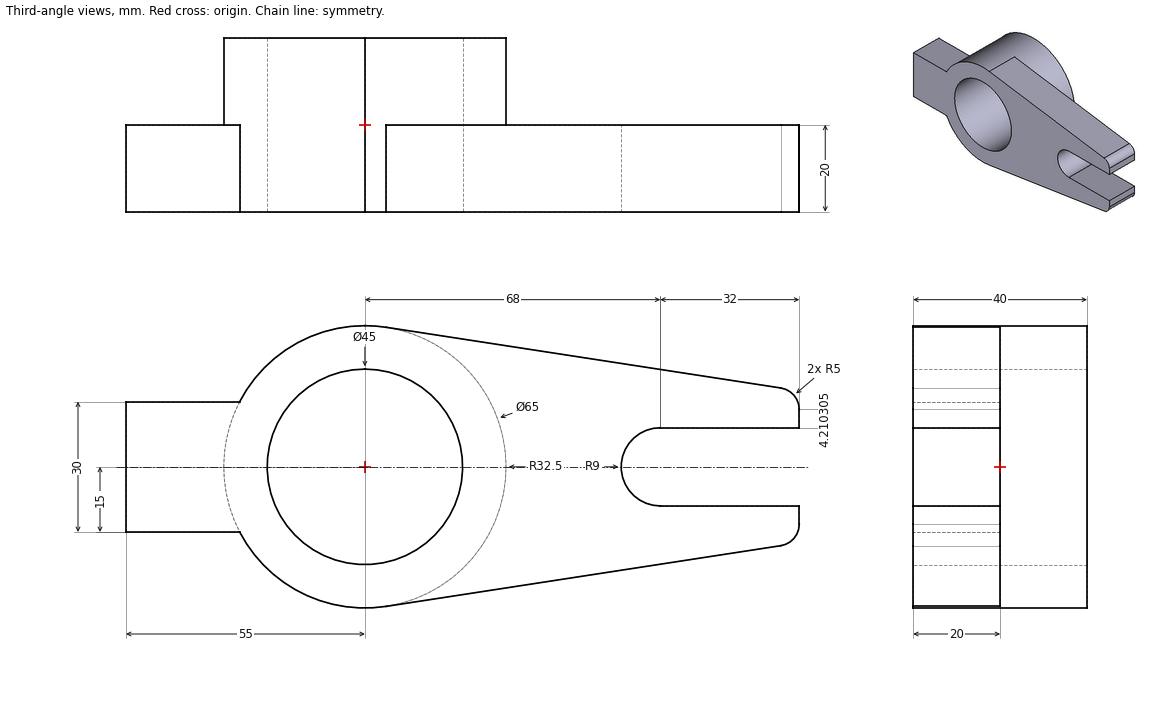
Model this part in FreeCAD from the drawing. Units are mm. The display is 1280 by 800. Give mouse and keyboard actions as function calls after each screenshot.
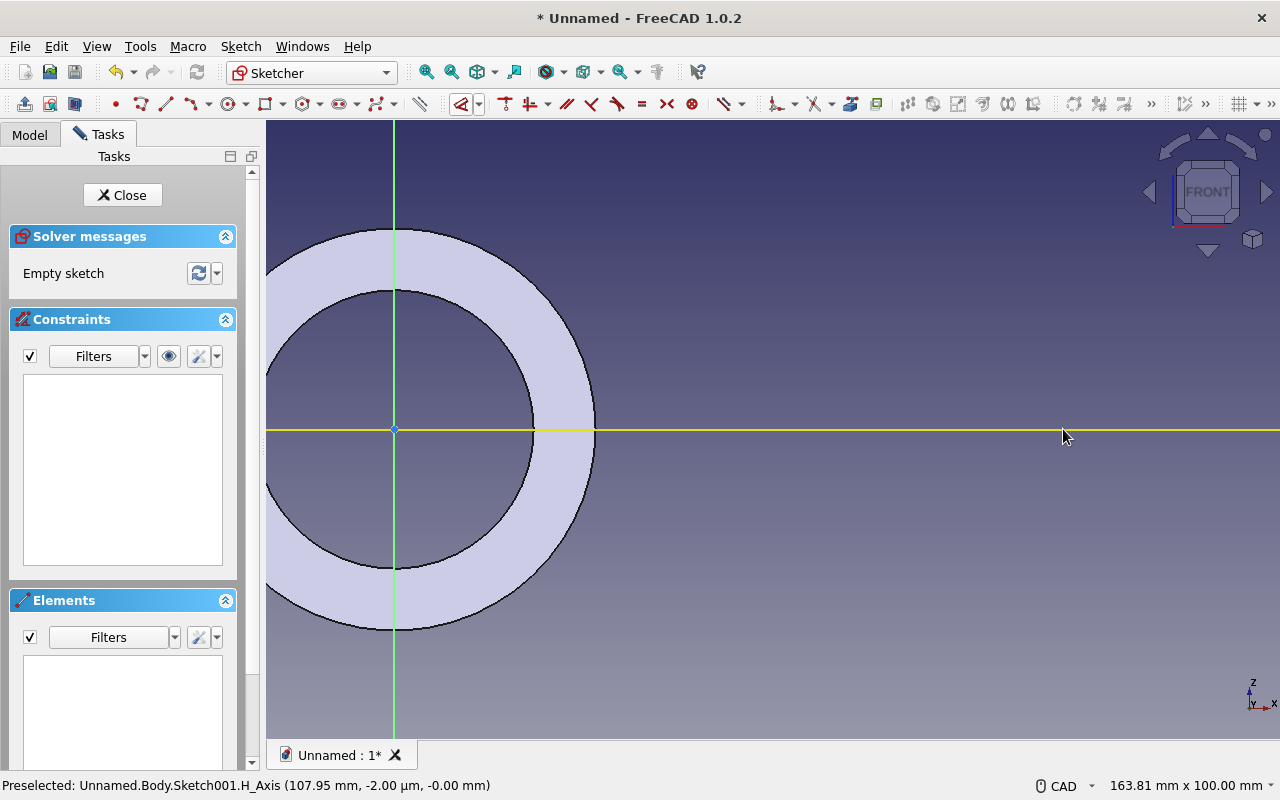
key(g)
key(l)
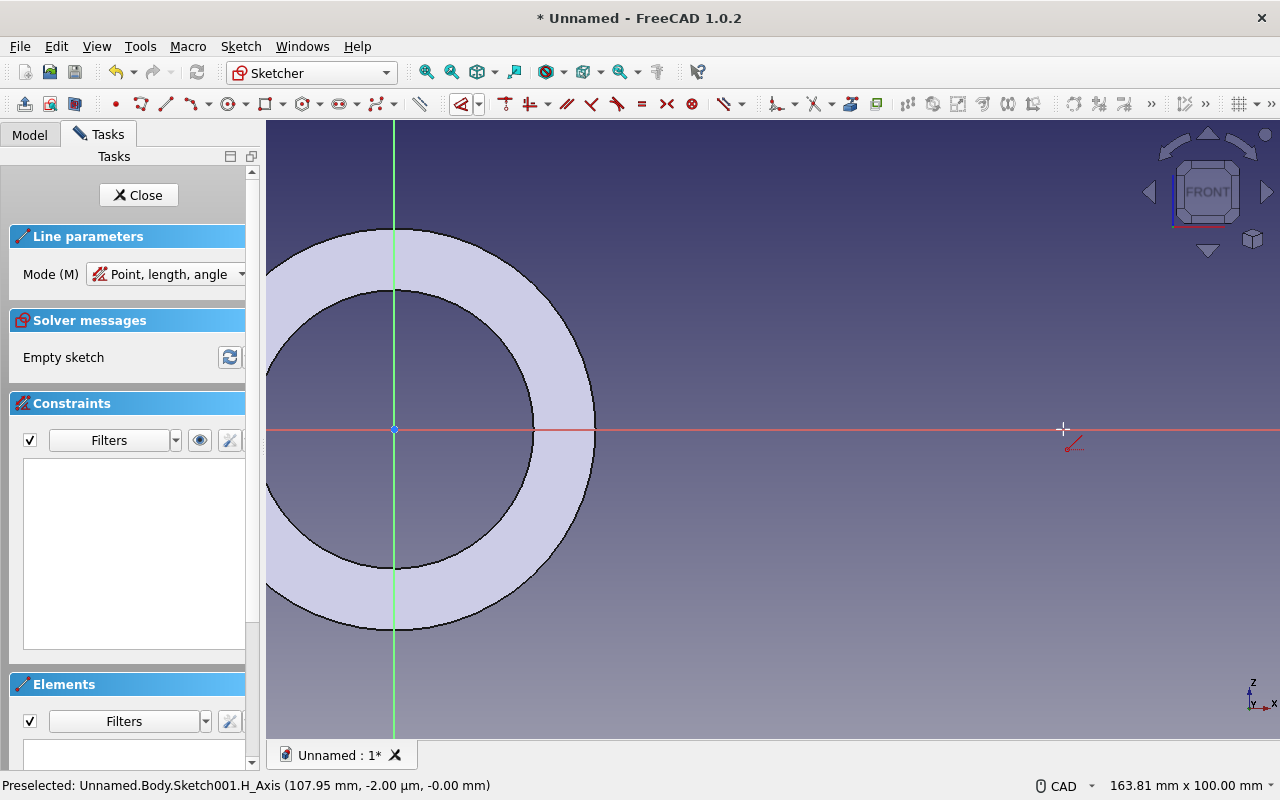
click(987, 542)
click(425, 628)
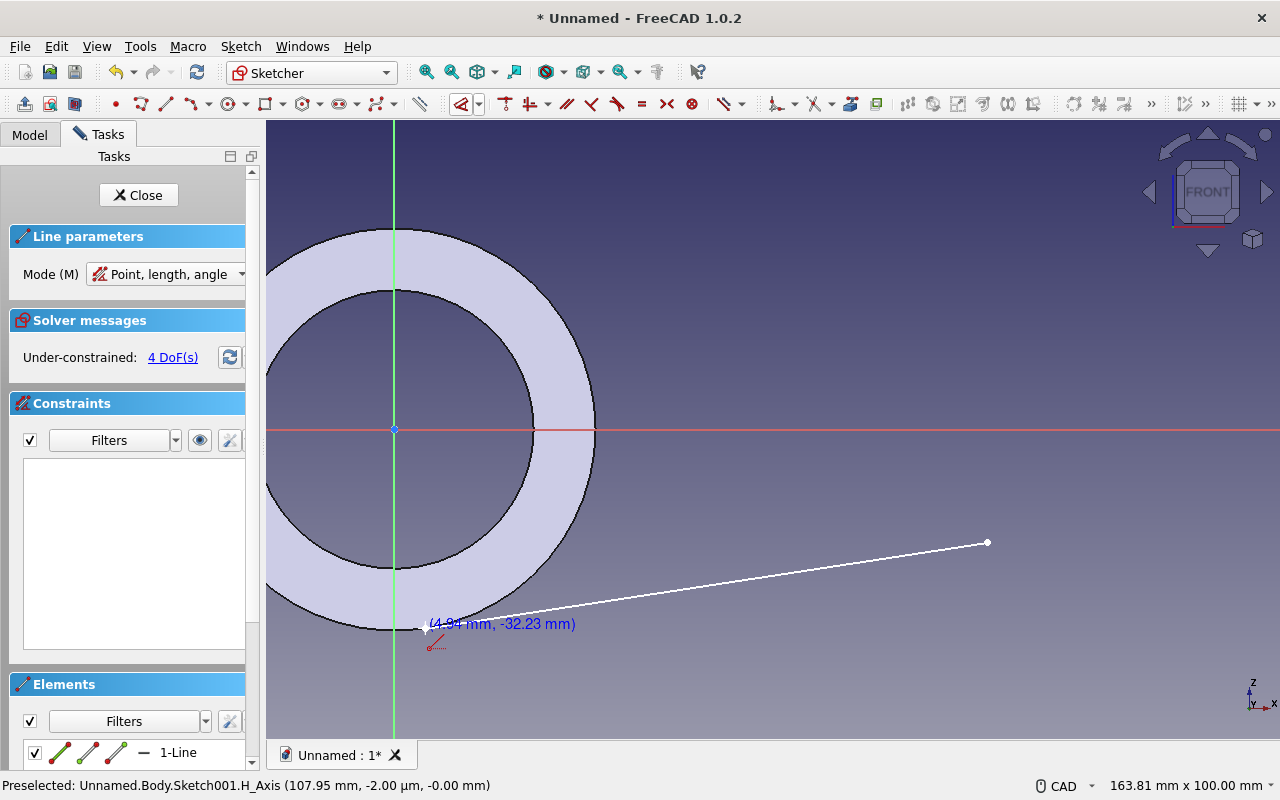
click(425, 231)
click(987, 317)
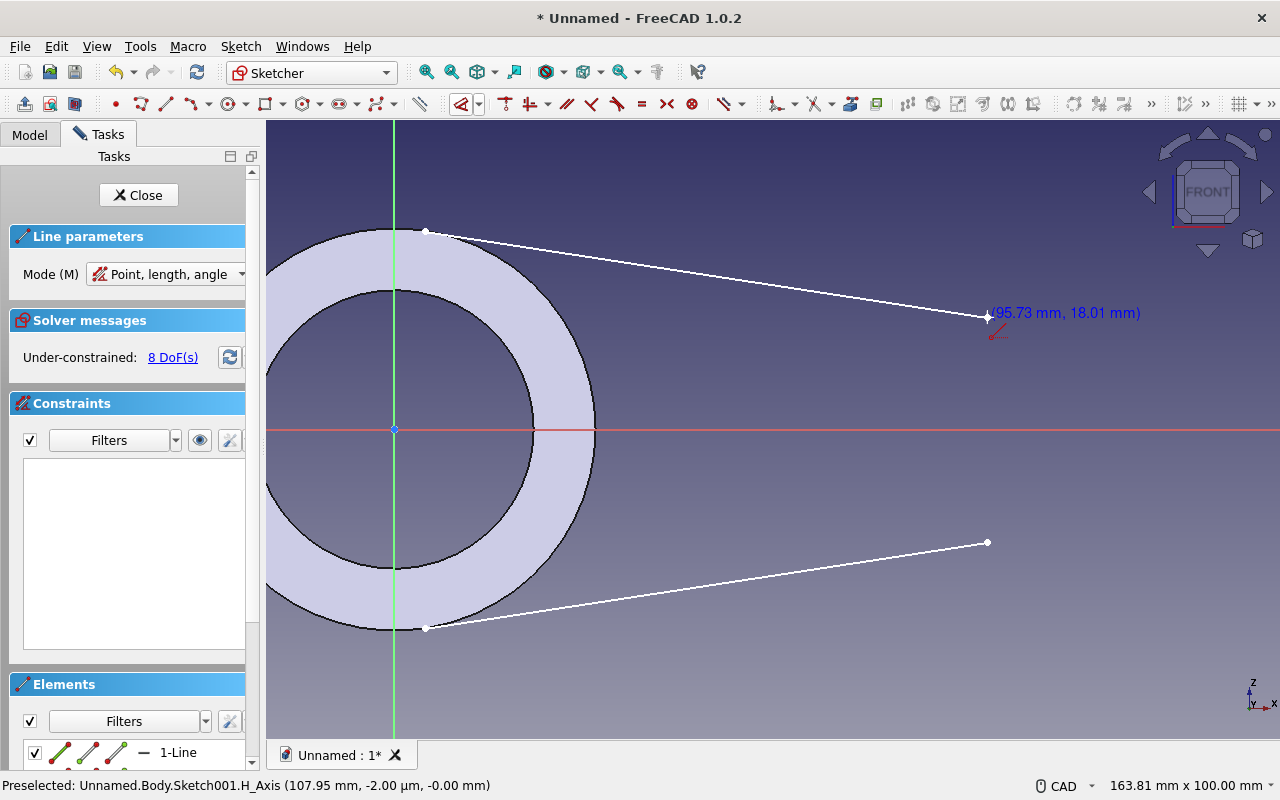
key(g)
key(m)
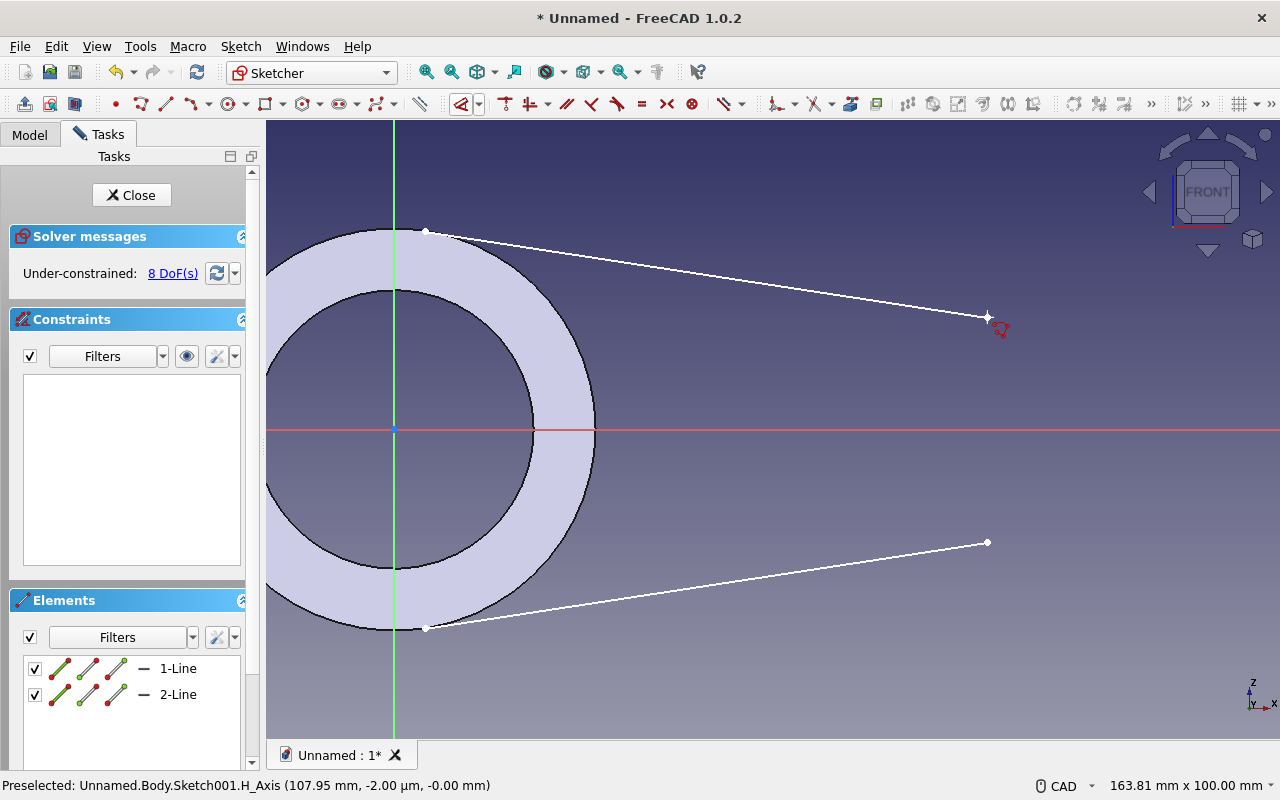
click(1013, 348)
click(1013, 374)
click(815, 374)
right_click(815, 374)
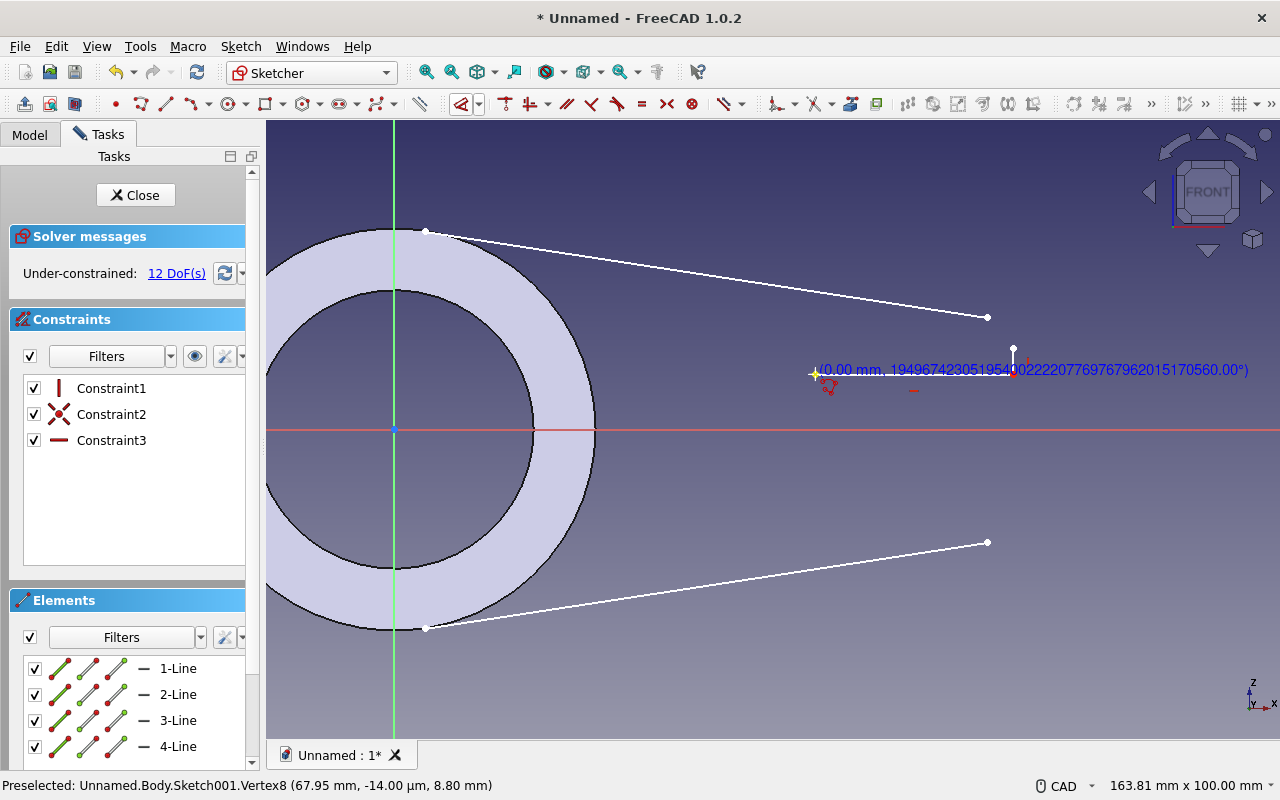
click(815, 485)
click(1013, 485)
click(1013, 511)
right_click(1013, 511)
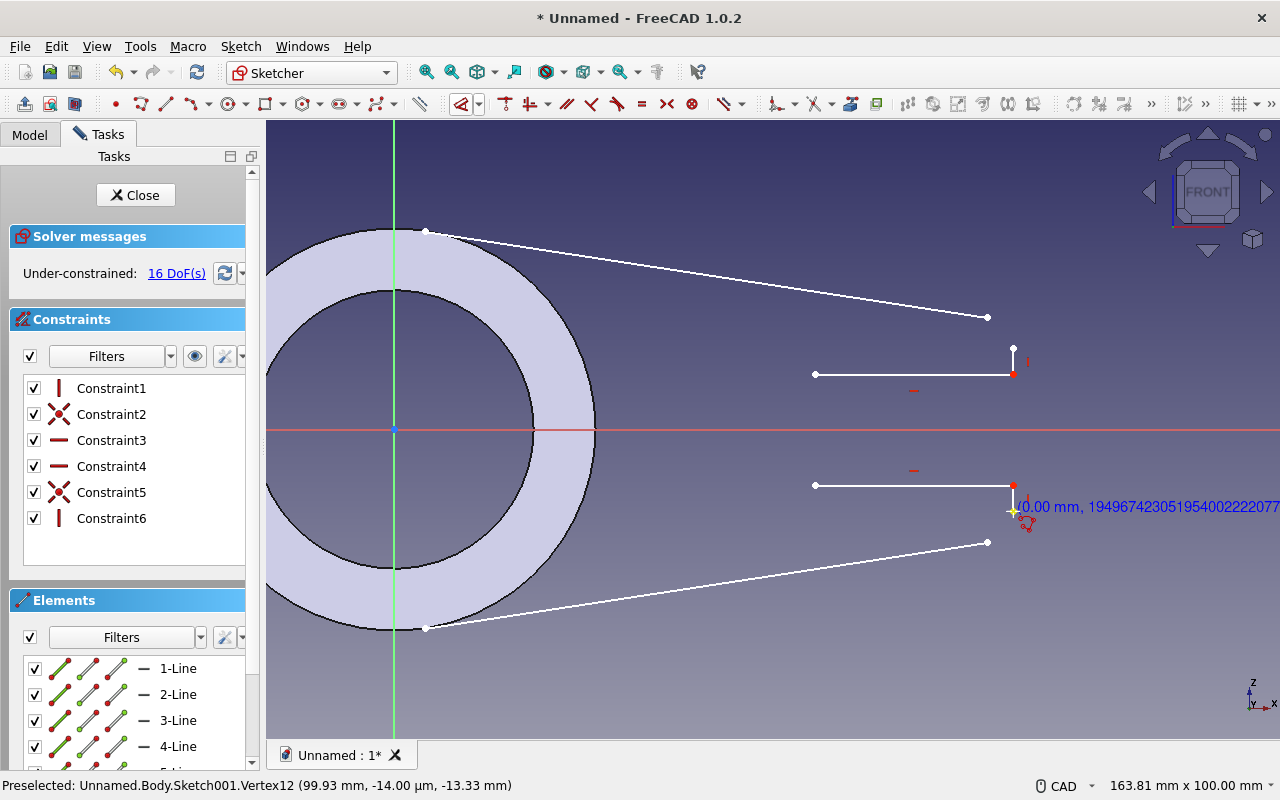
key(g)
key(3)
key(a)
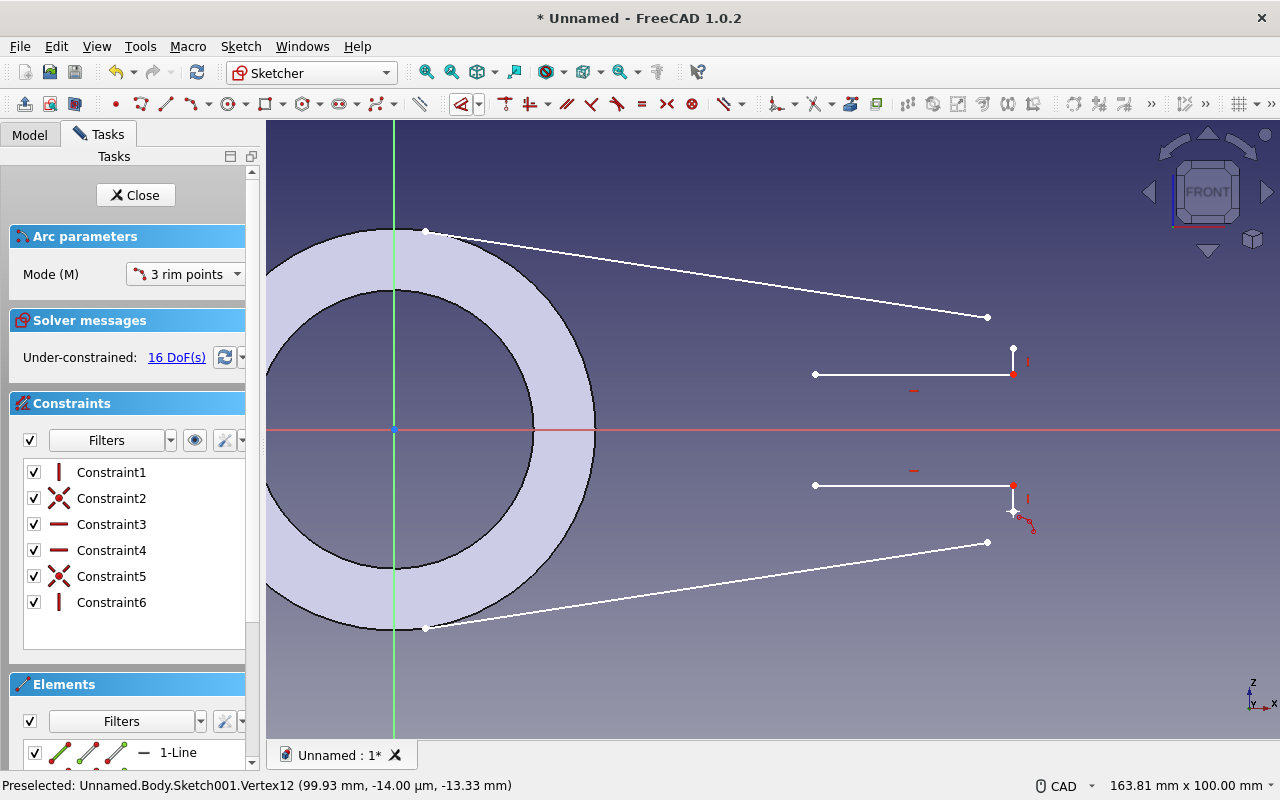
click(425, 629)
click(425, 232)
click(588, 486)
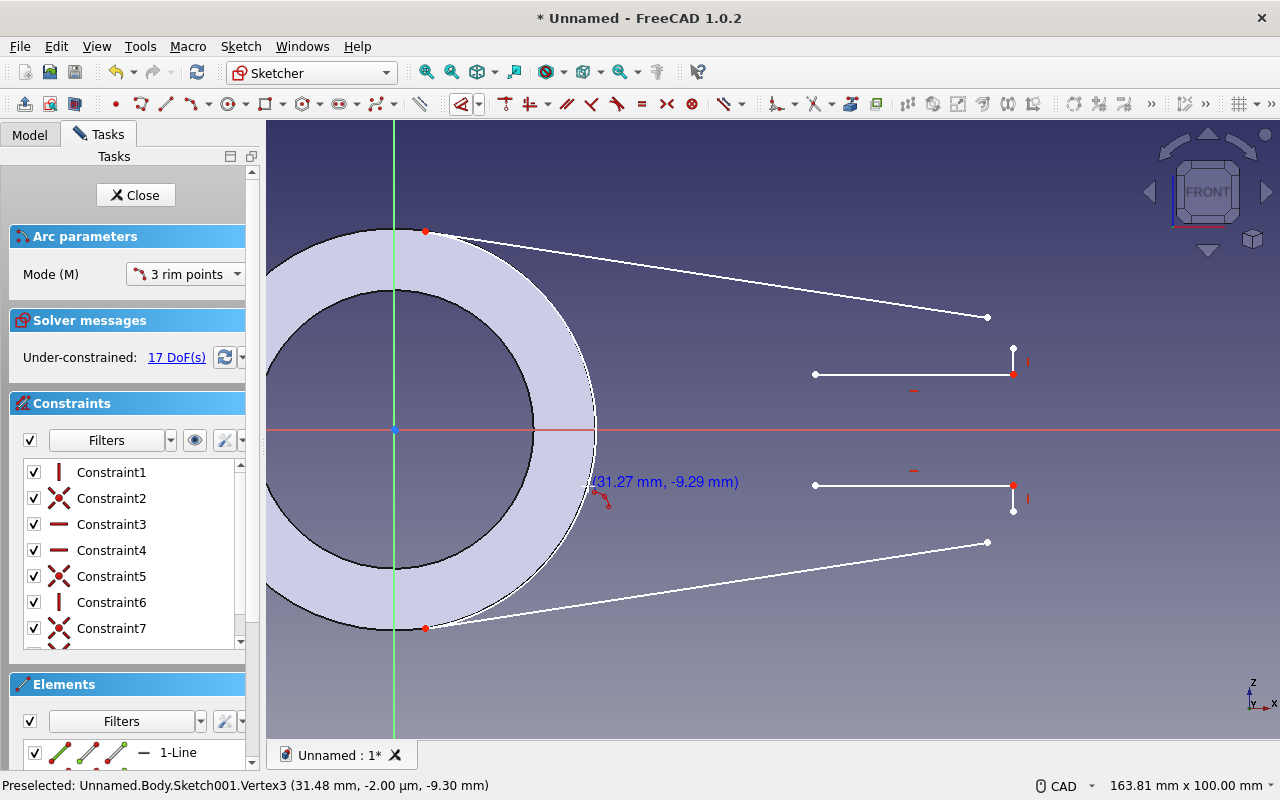
click(987, 318)
click(1013, 349)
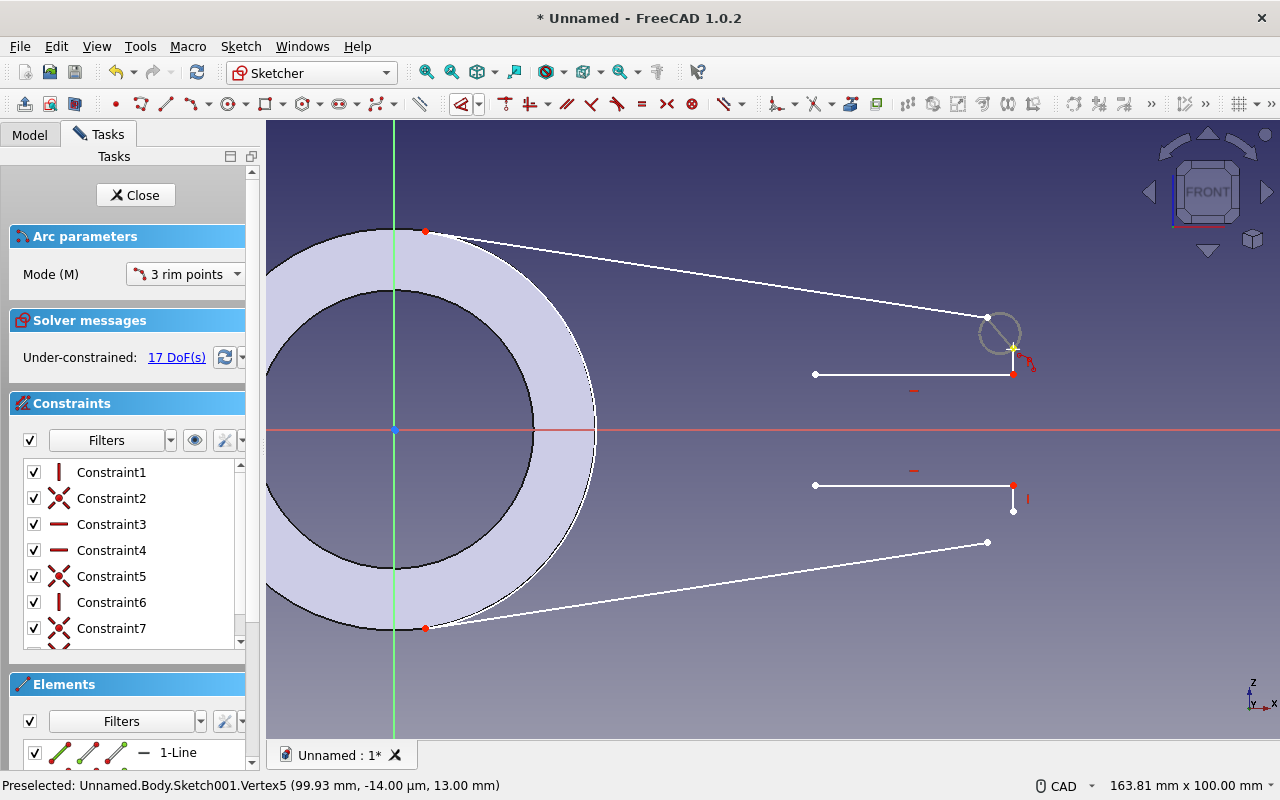
scroll(1006, 328, up, 4)